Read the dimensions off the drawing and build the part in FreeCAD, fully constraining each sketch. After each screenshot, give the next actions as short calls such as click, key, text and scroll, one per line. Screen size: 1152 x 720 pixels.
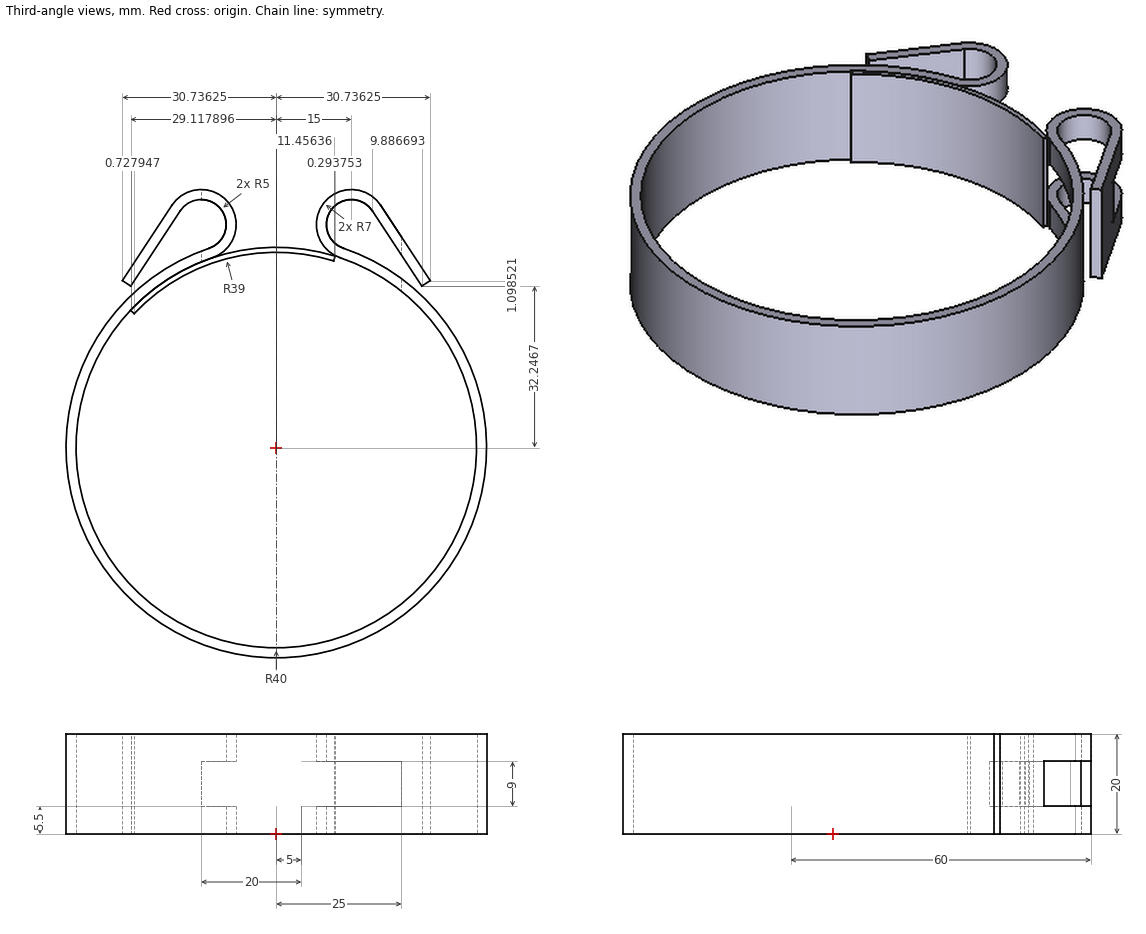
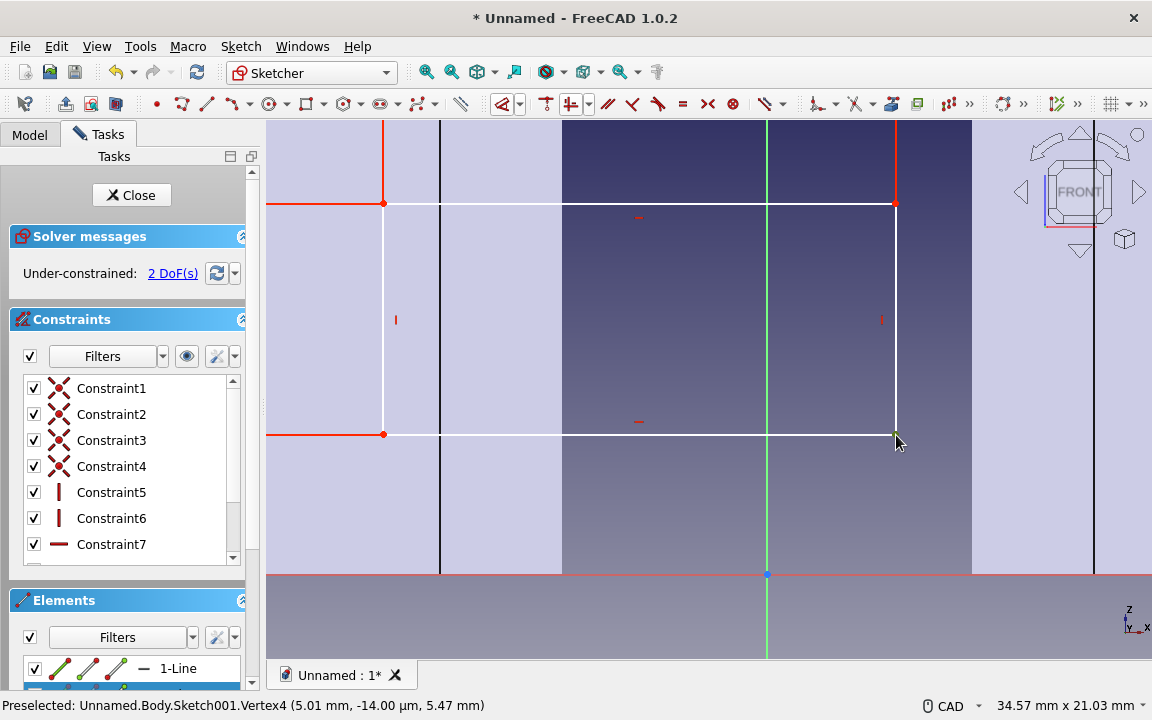
key(l)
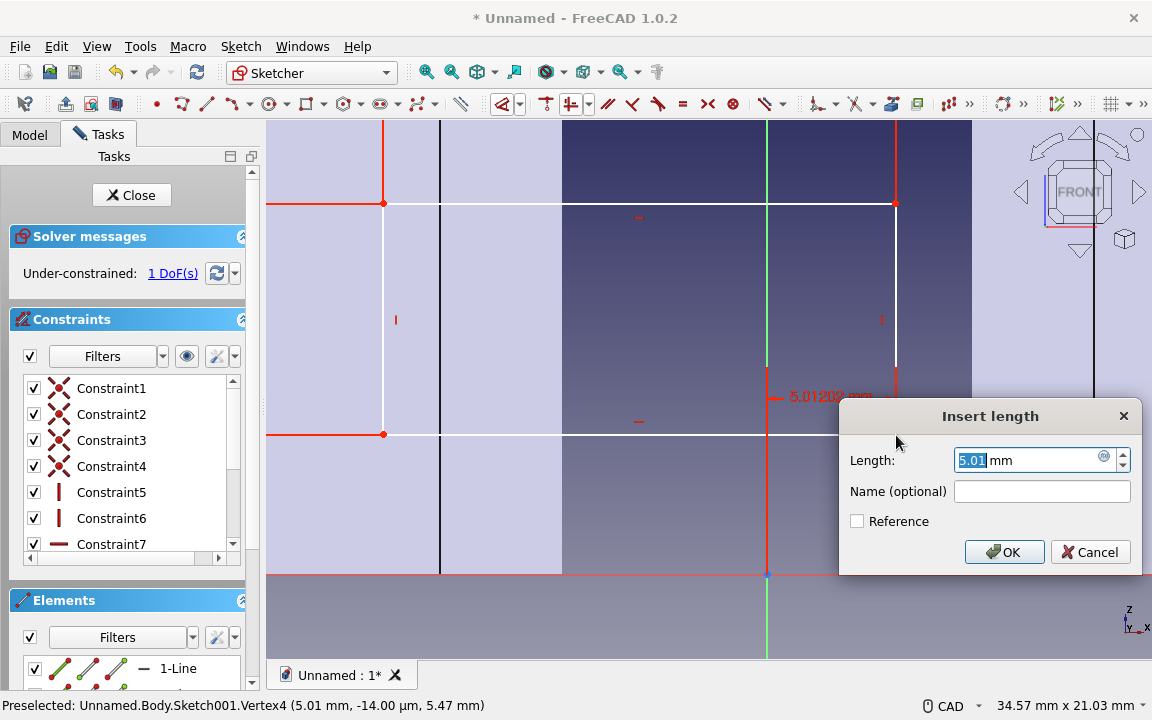
text(5)
key(Return)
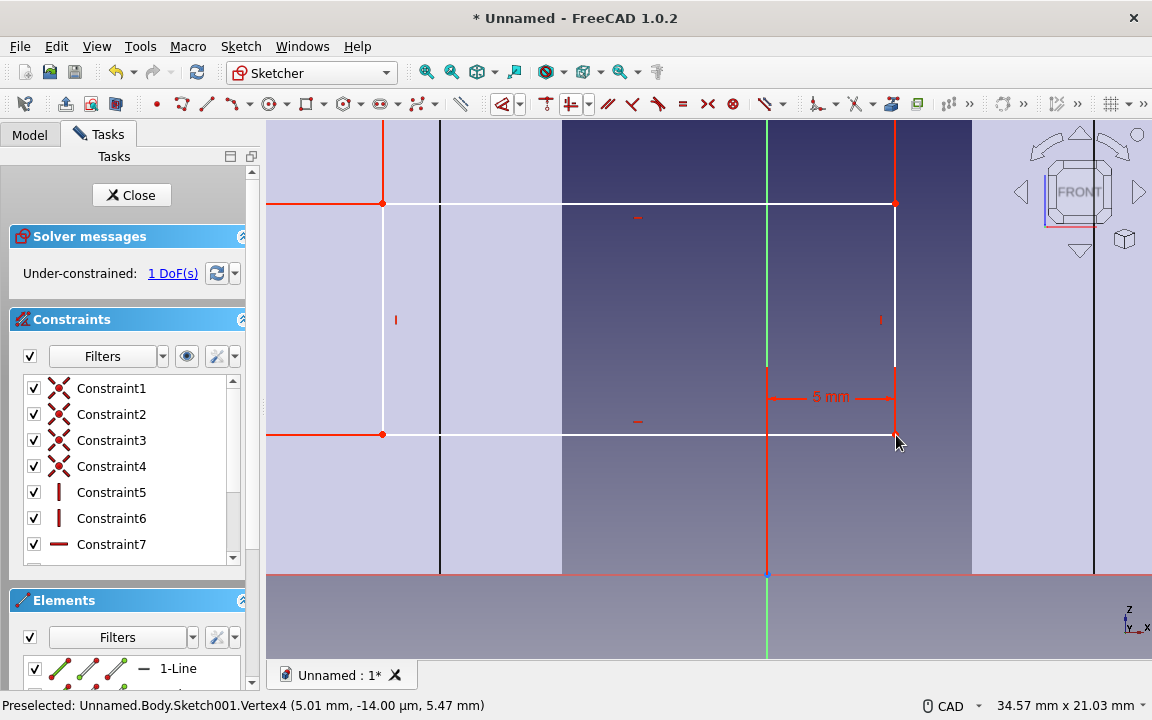
click(383, 435)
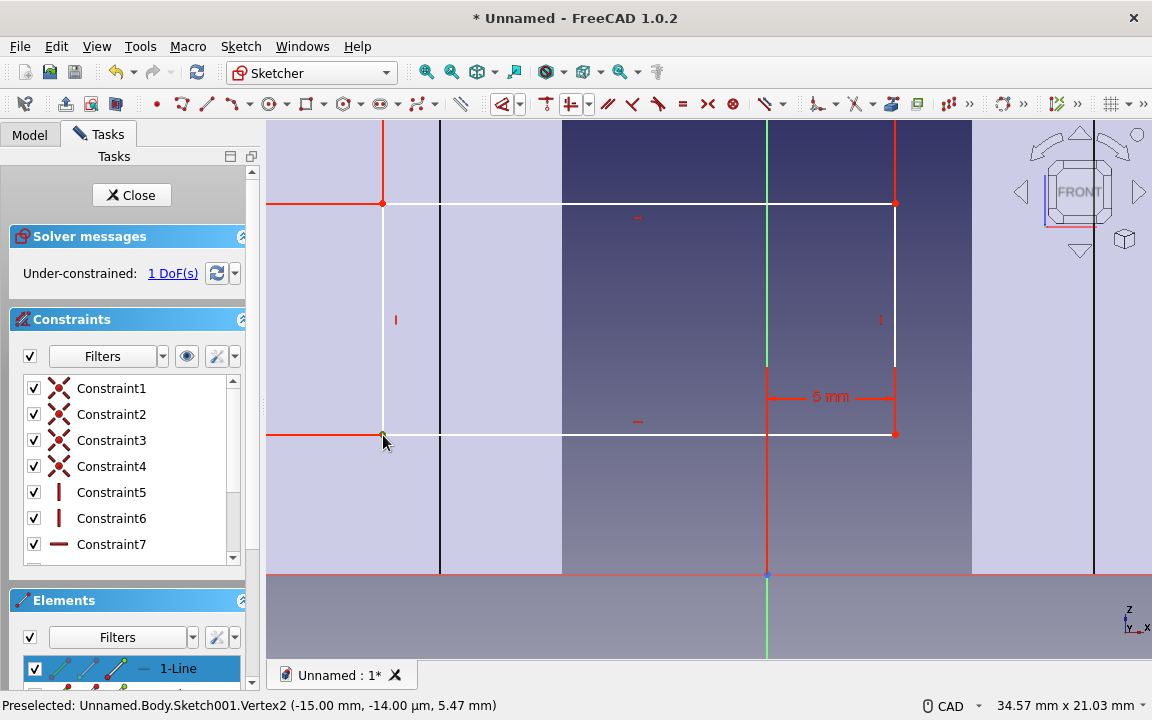
key(i)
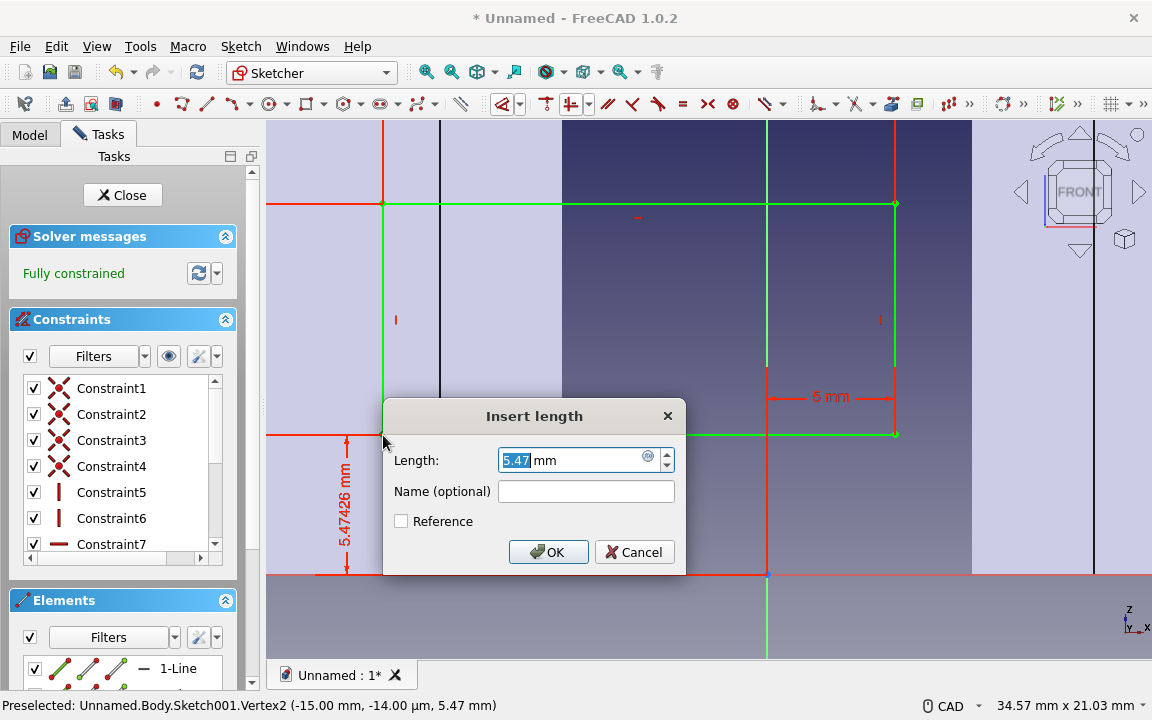
text(5.5)
key(Return)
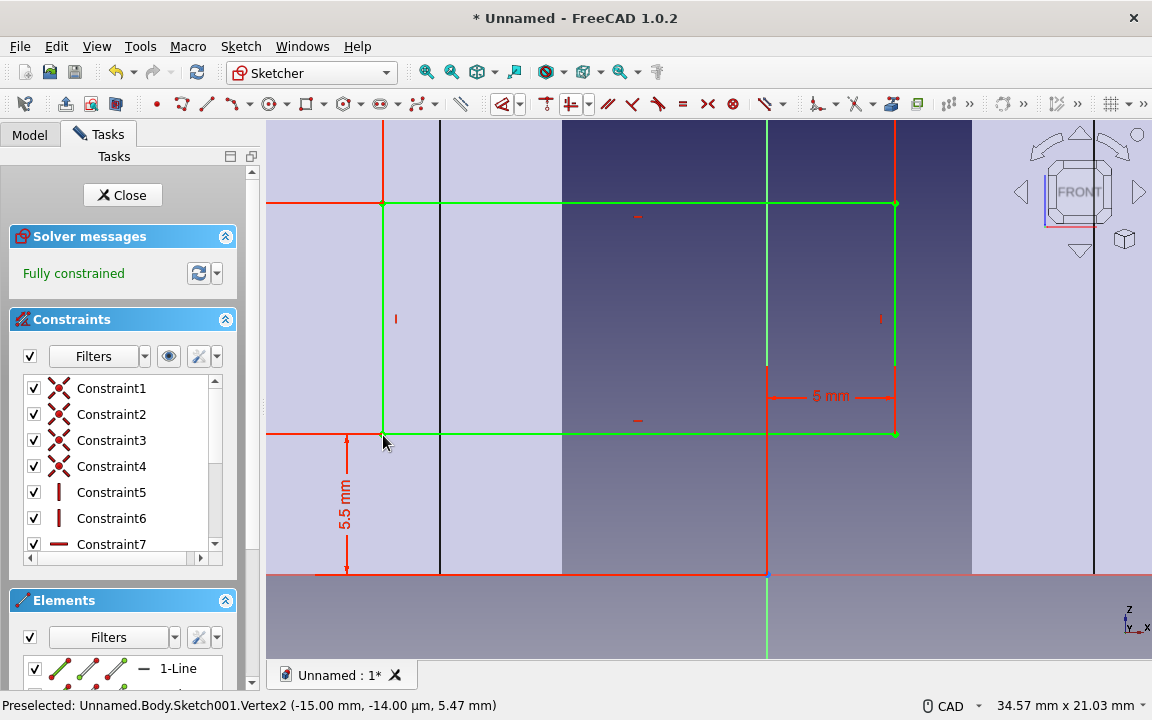
click(123, 195)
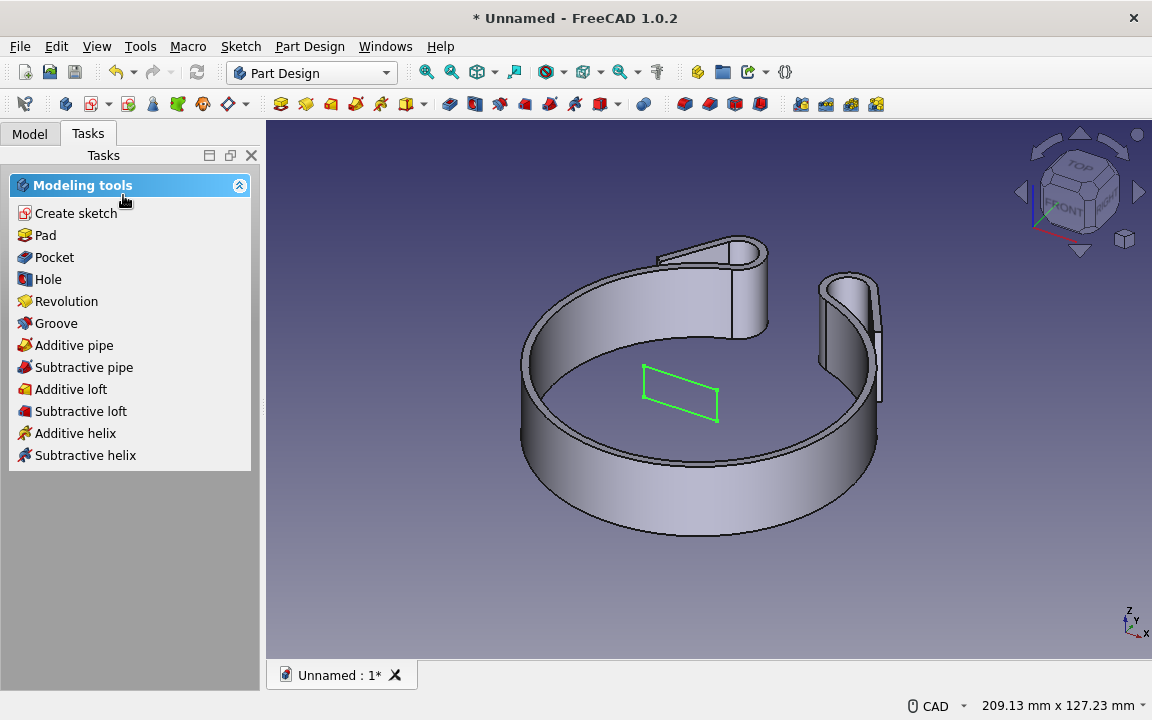
click(450, 104)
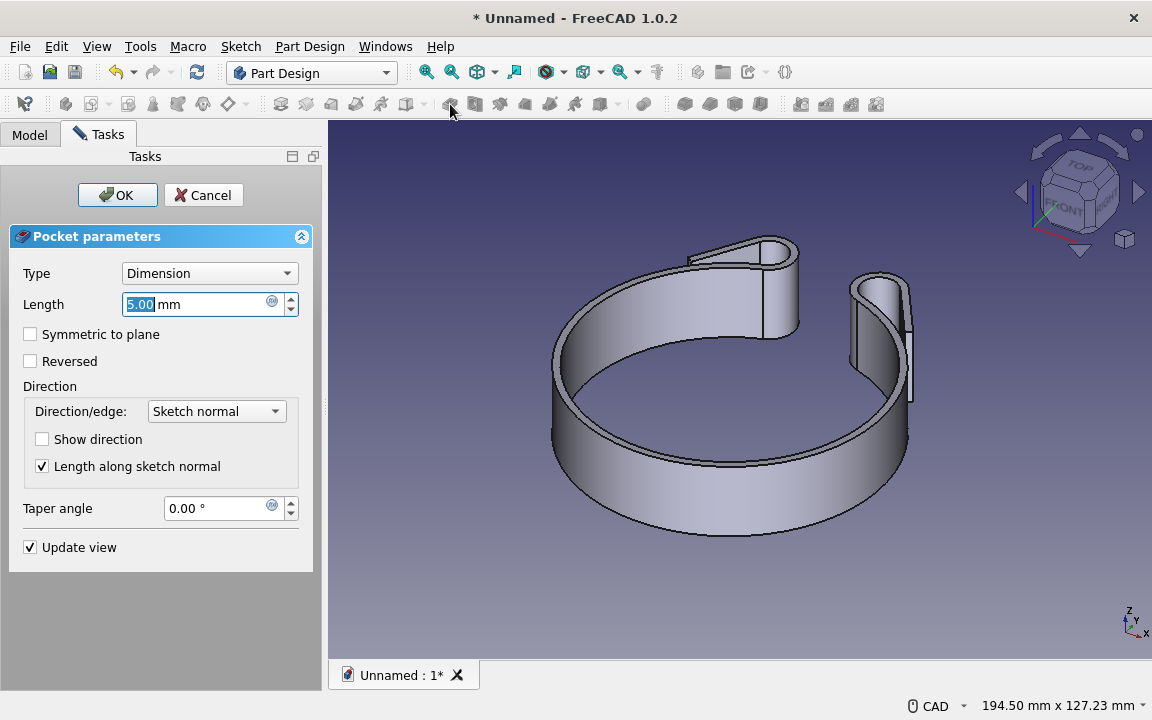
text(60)
key(Tab)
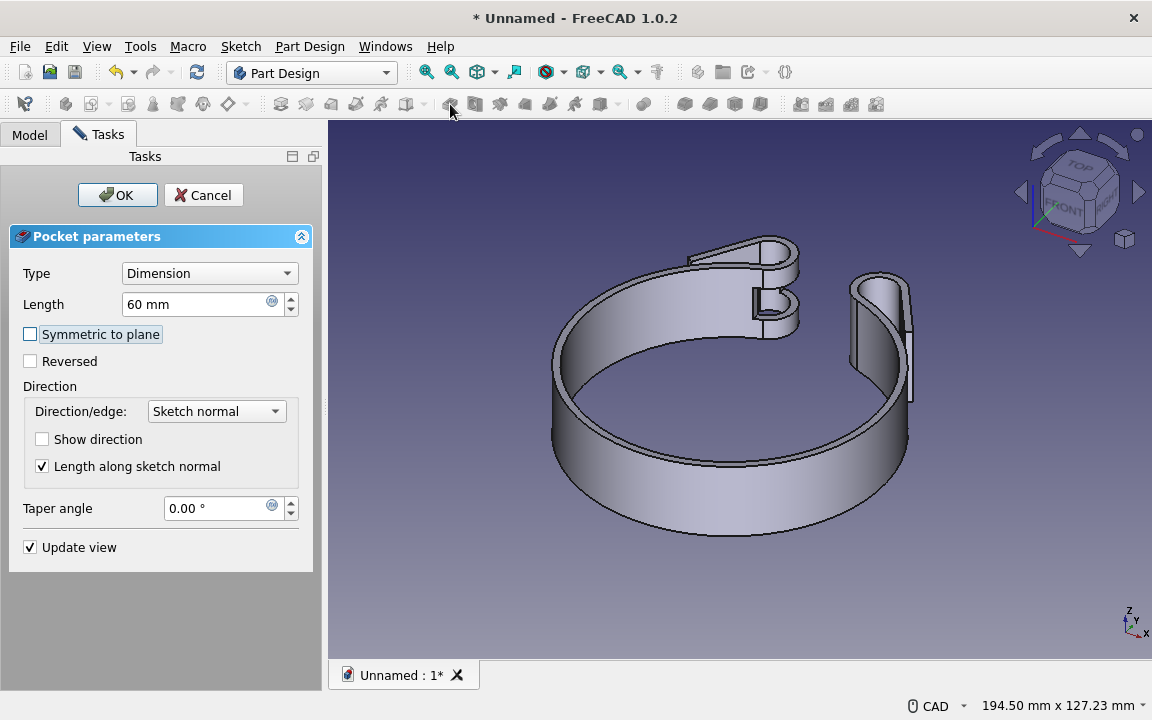
click(118, 195)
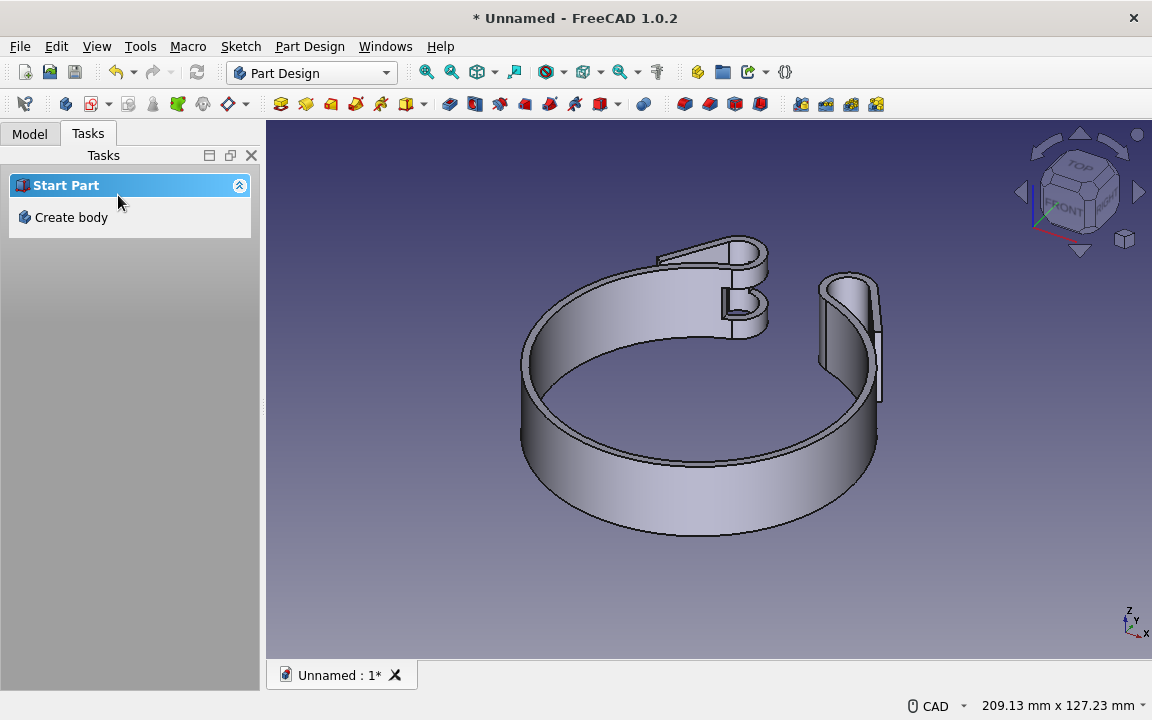
click(30, 134)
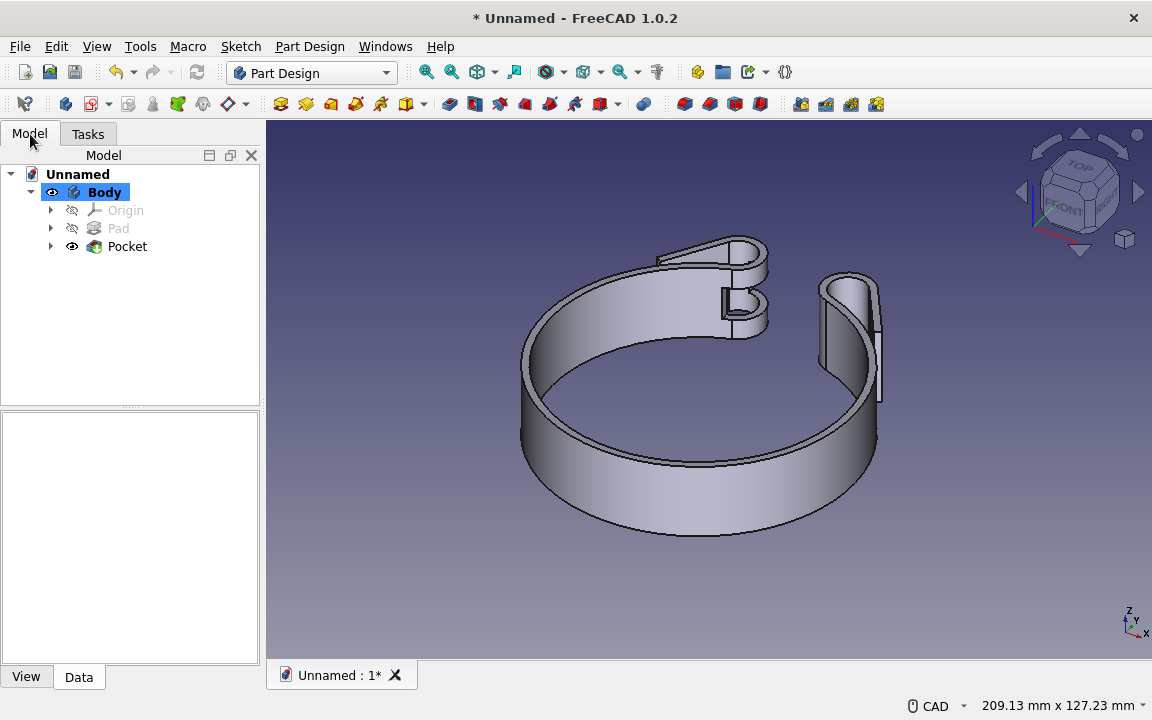
click(51, 210)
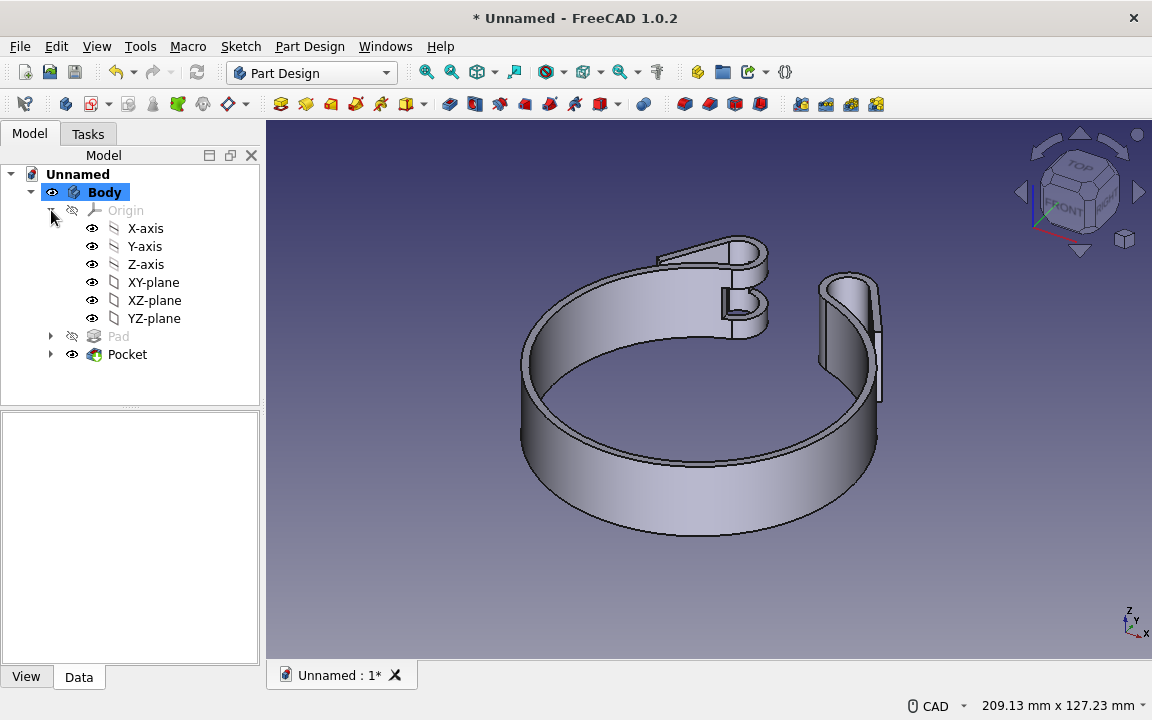
click(137, 300)